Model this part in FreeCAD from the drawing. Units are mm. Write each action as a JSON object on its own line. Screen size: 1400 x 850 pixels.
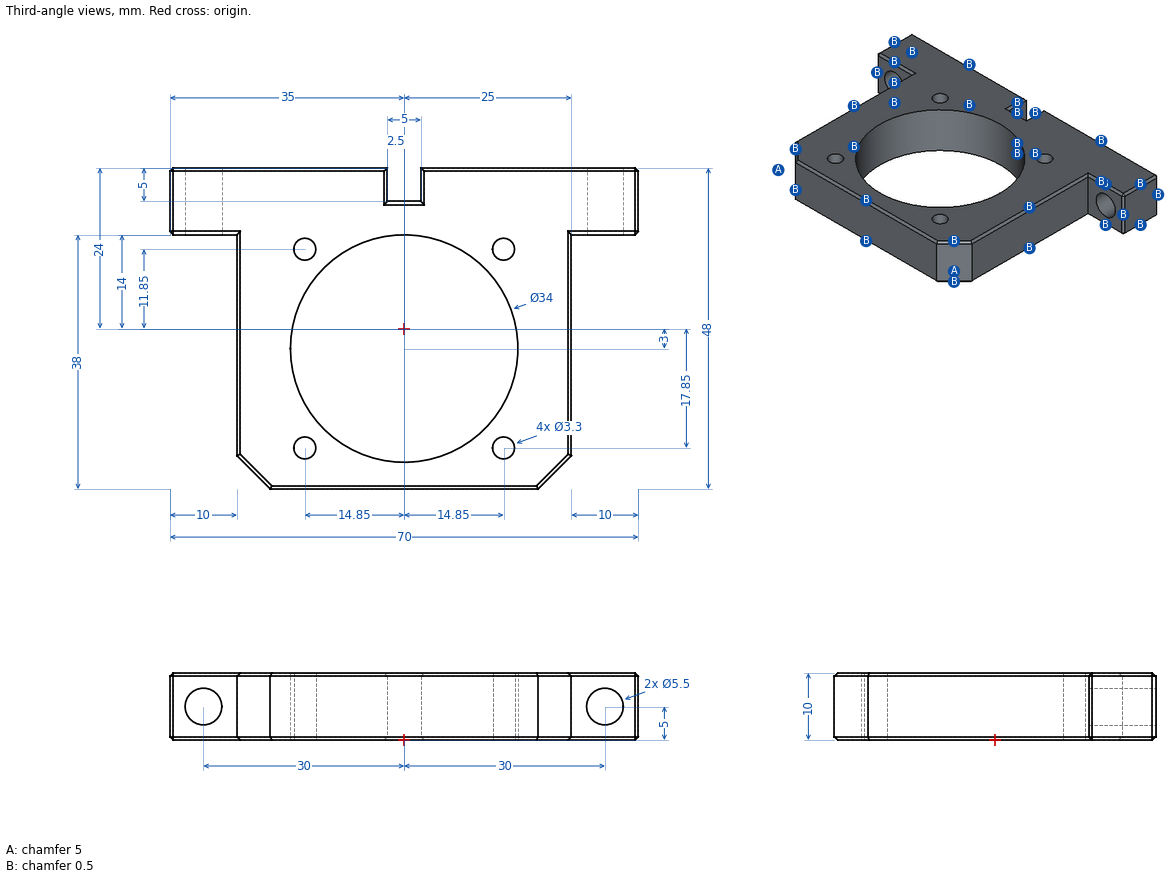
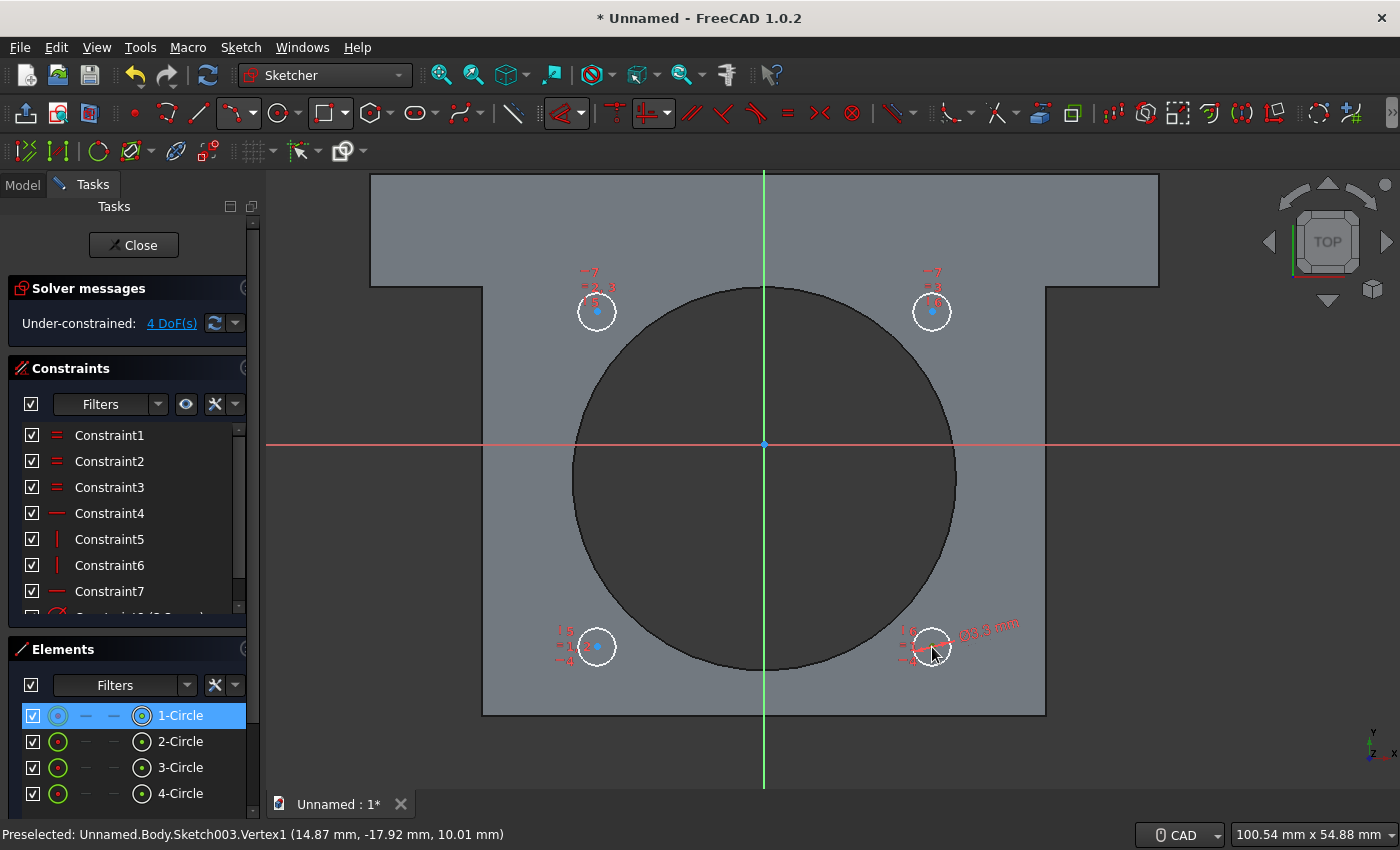
{"action": "left_click", "coordinate": [584, 114]}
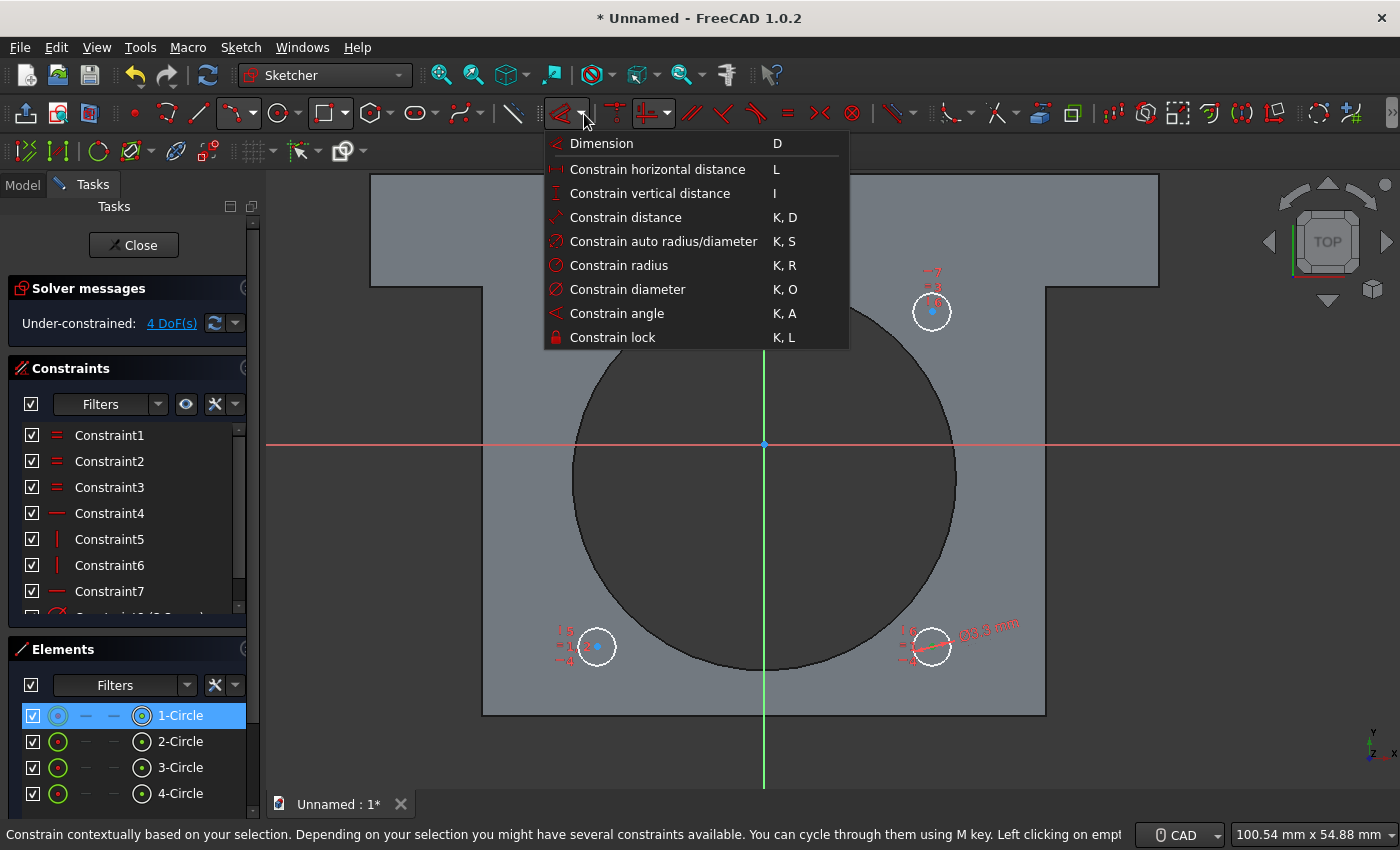
{"action": "left_click", "coordinate": [697, 169]}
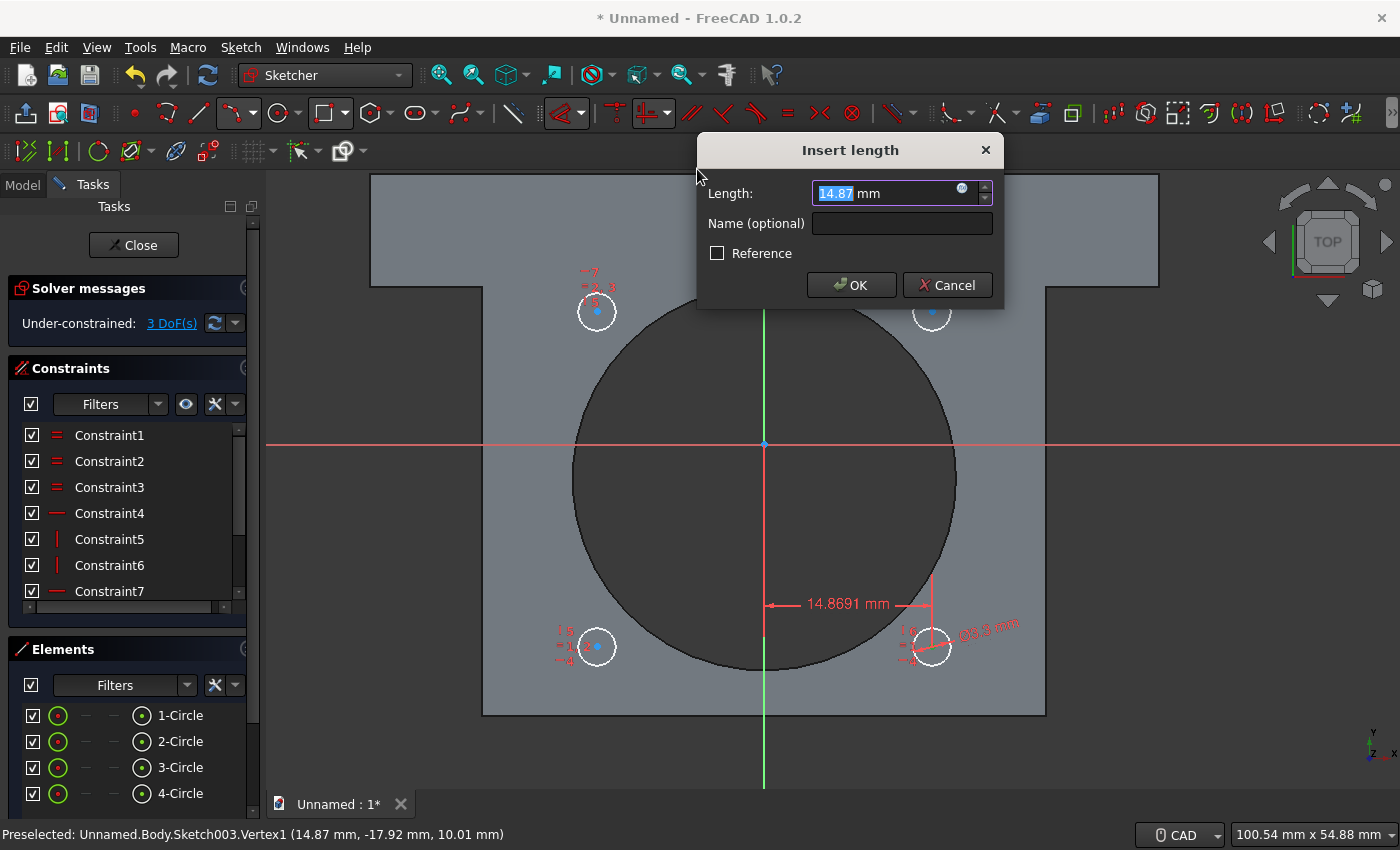
{"action": "type", "text": "14.85"}
{"action": "key", "text": "Return"}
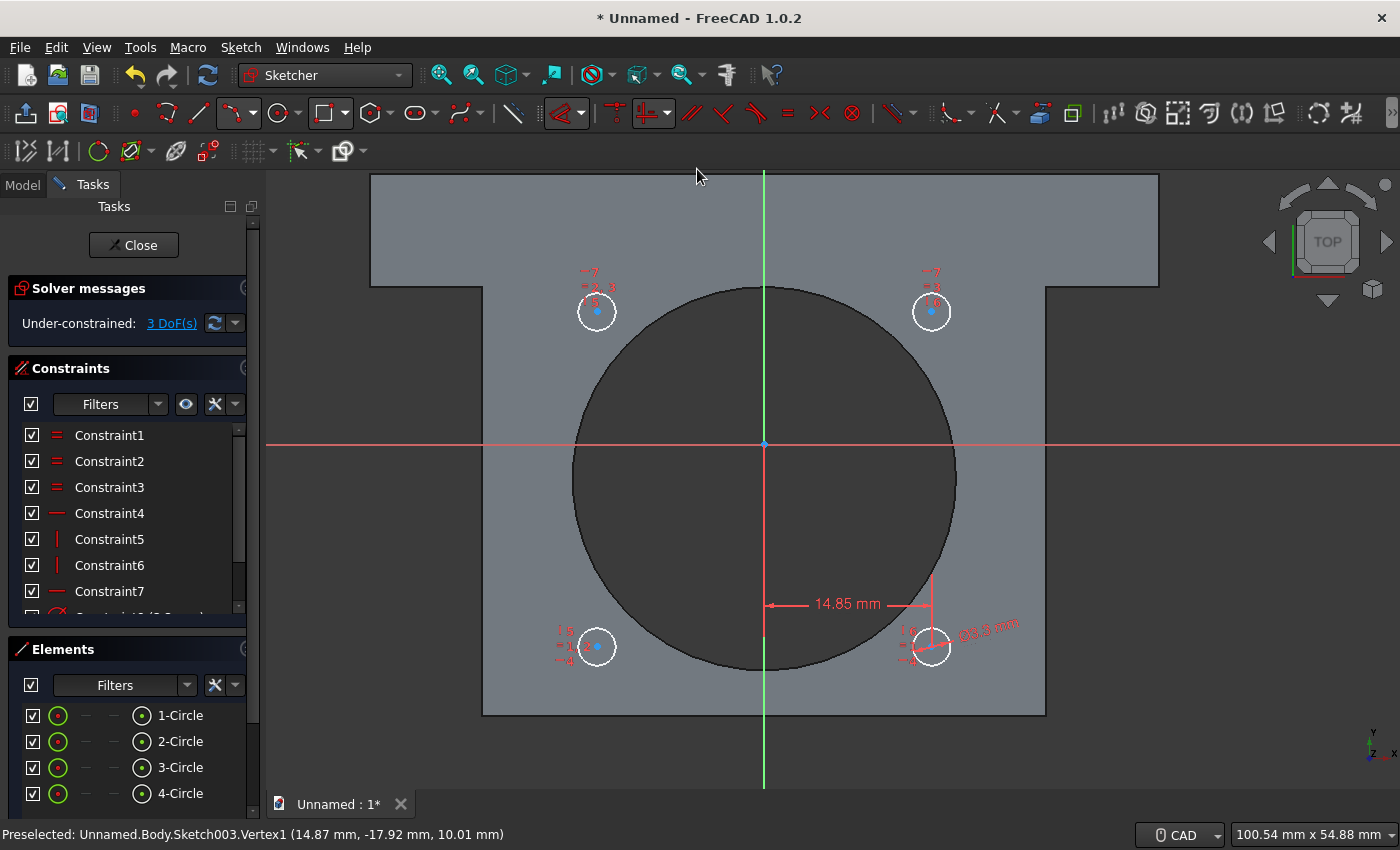
{"action": "left_click", "coordinate": [932, 647]}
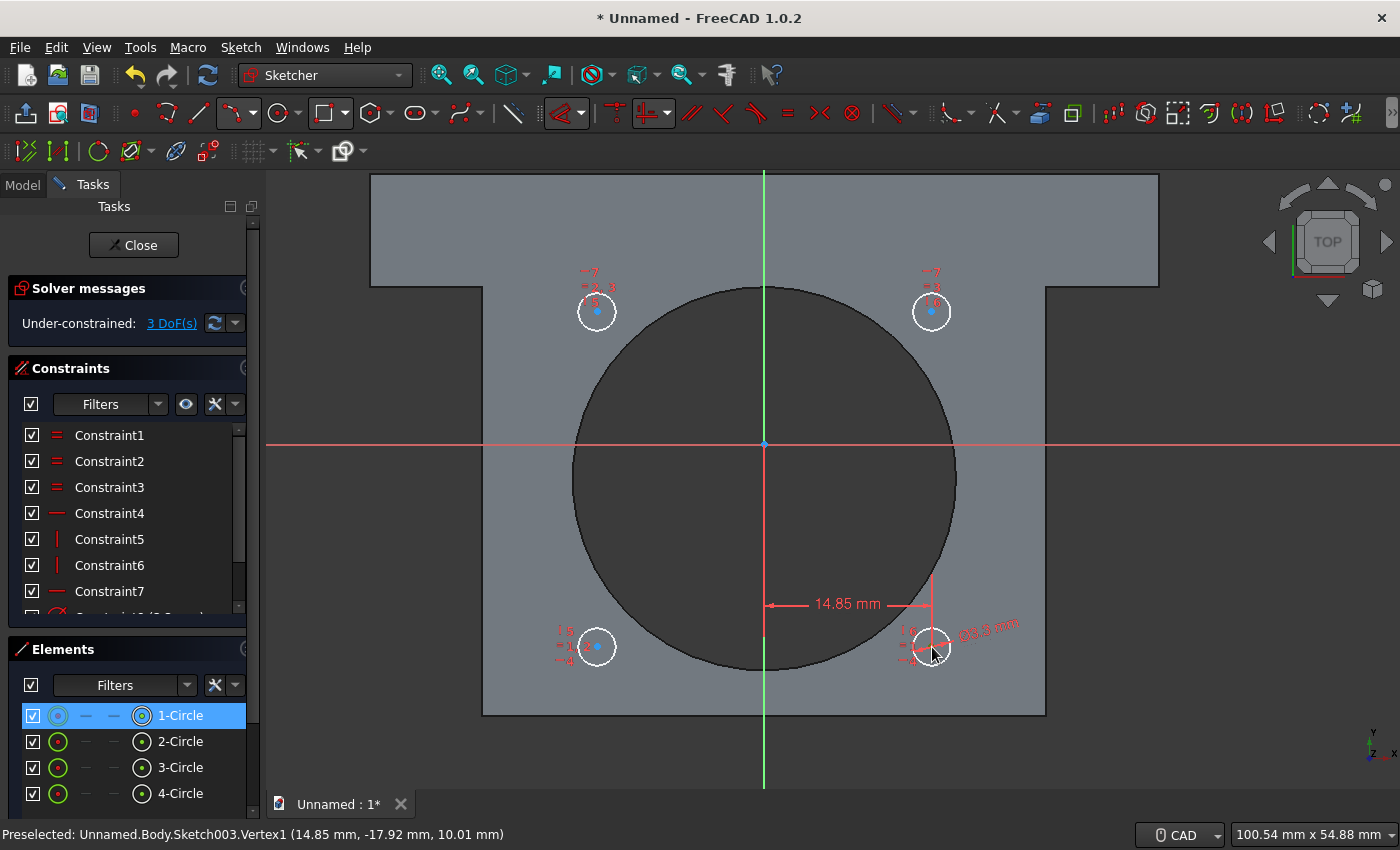
{"action": "key", "text": "i"}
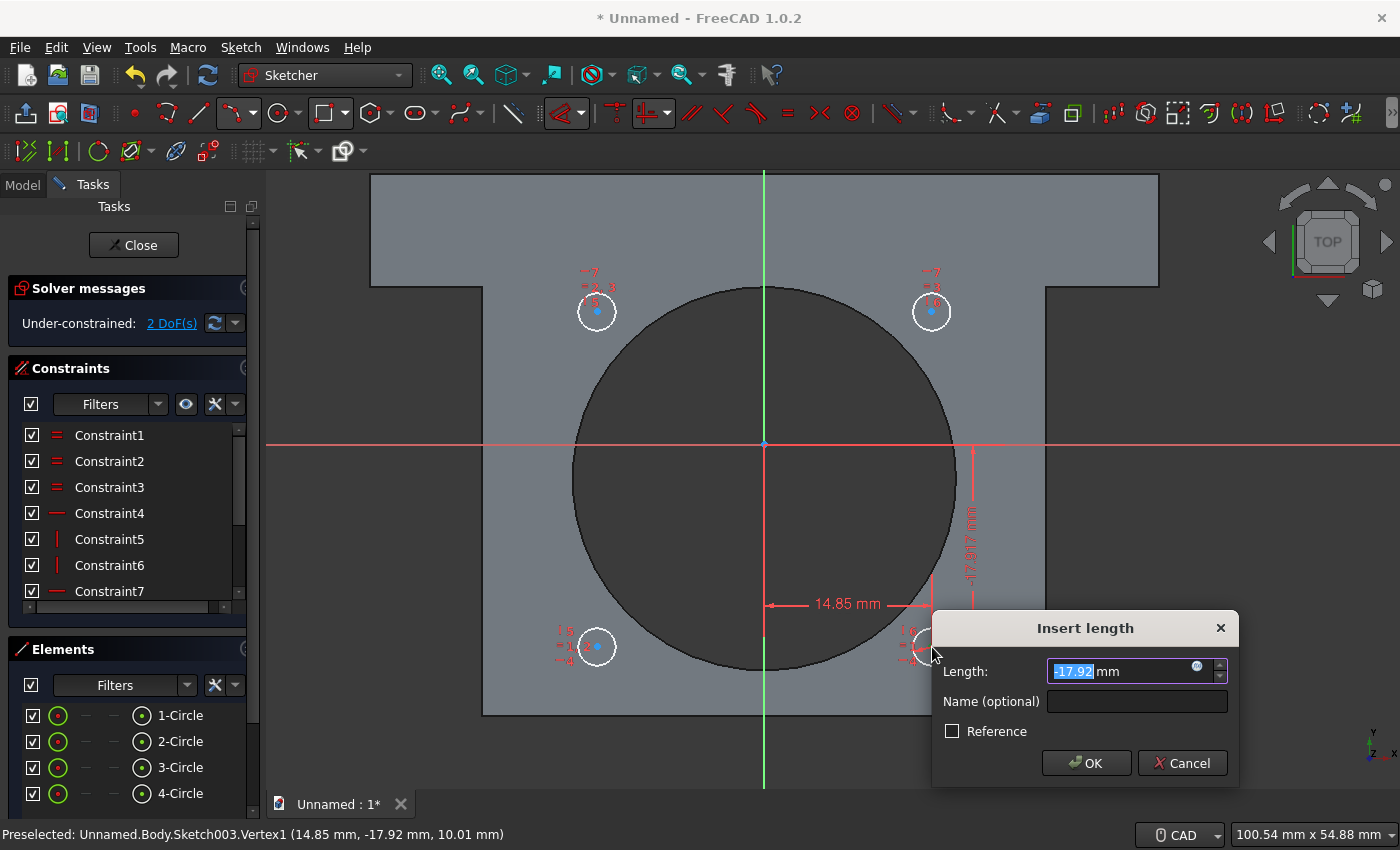
{"action": "type", "text": "-17.85"}
{"action": "key", "text": "Return"}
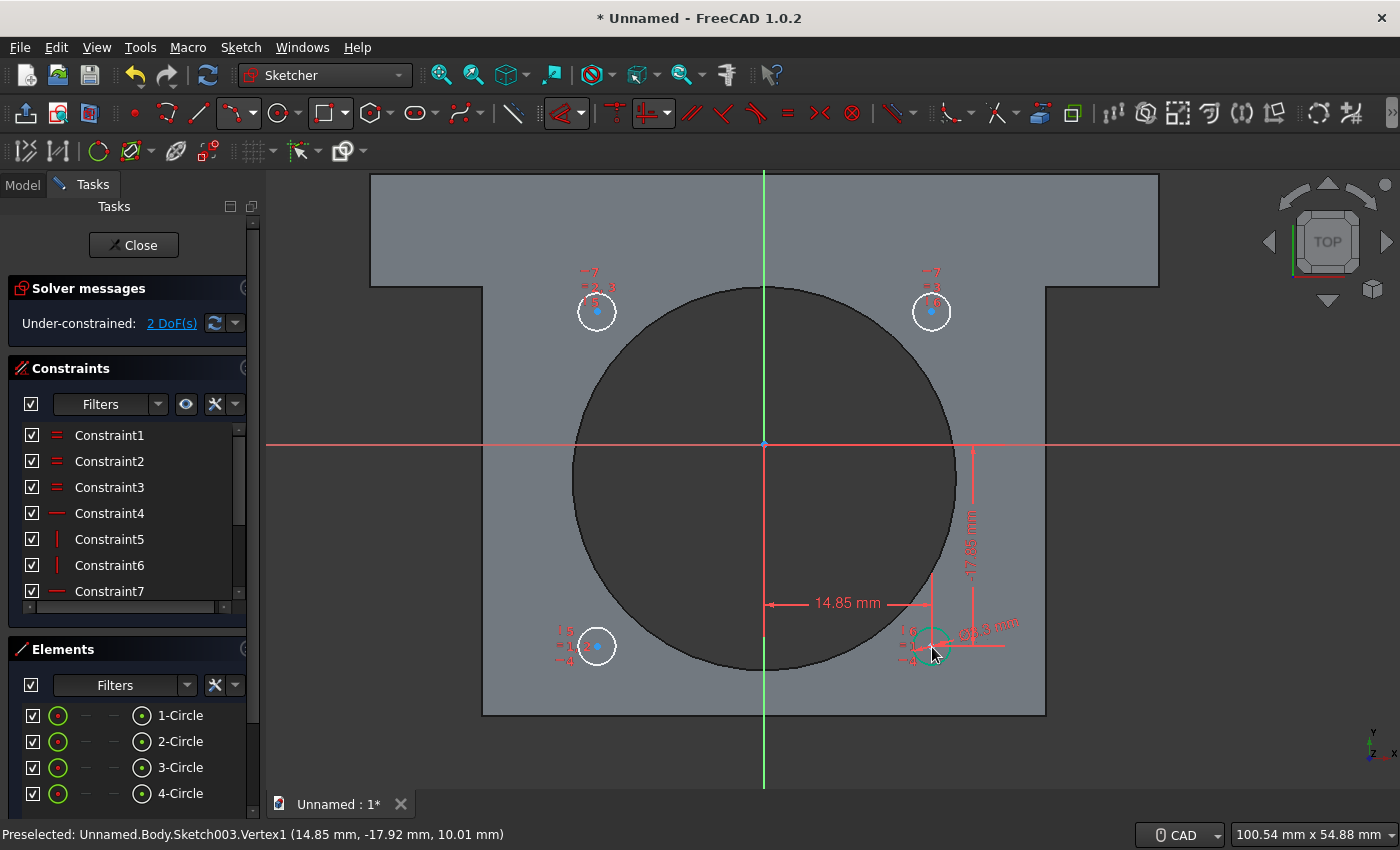
{"action": "left_click", "coordinate": [597, 646]}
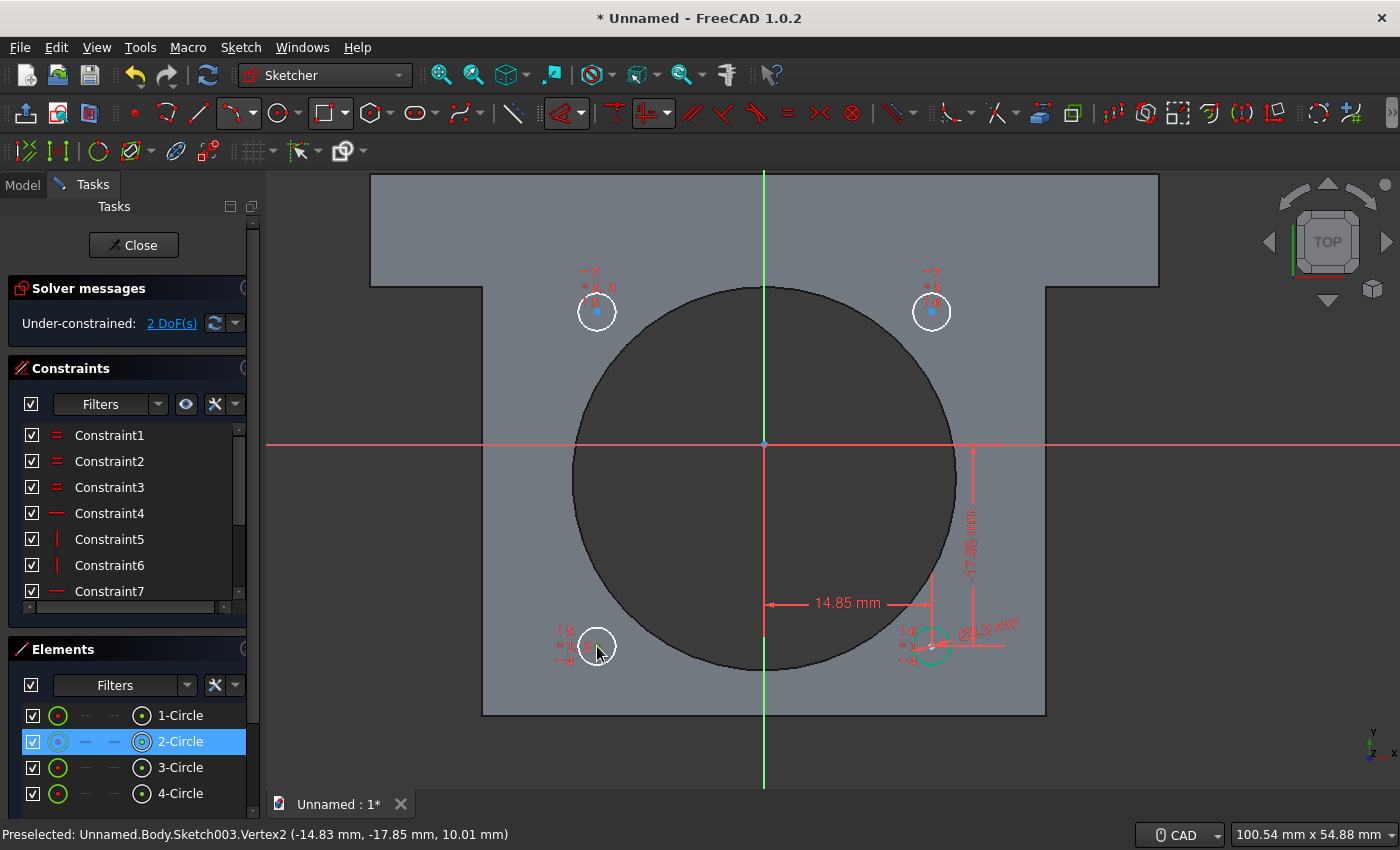
{"action": "key", "text": "l"}